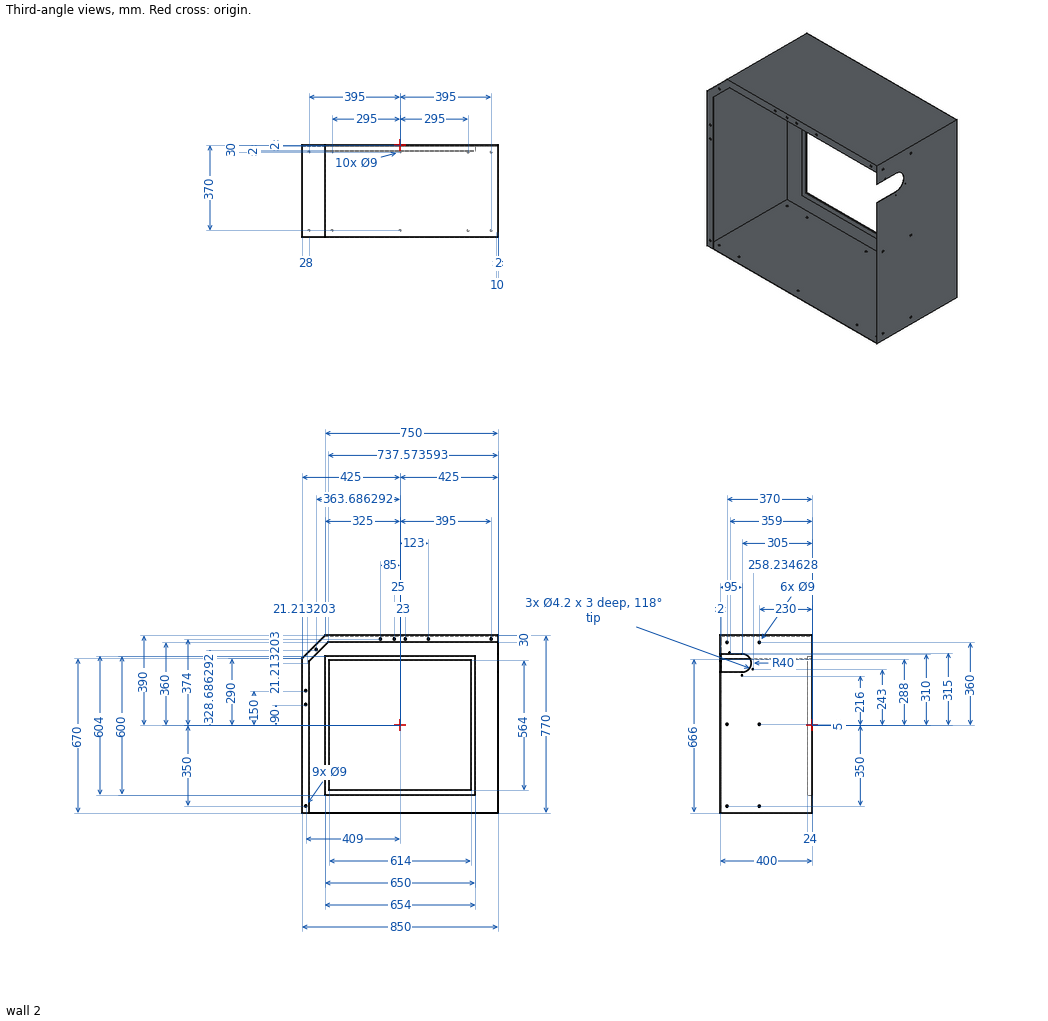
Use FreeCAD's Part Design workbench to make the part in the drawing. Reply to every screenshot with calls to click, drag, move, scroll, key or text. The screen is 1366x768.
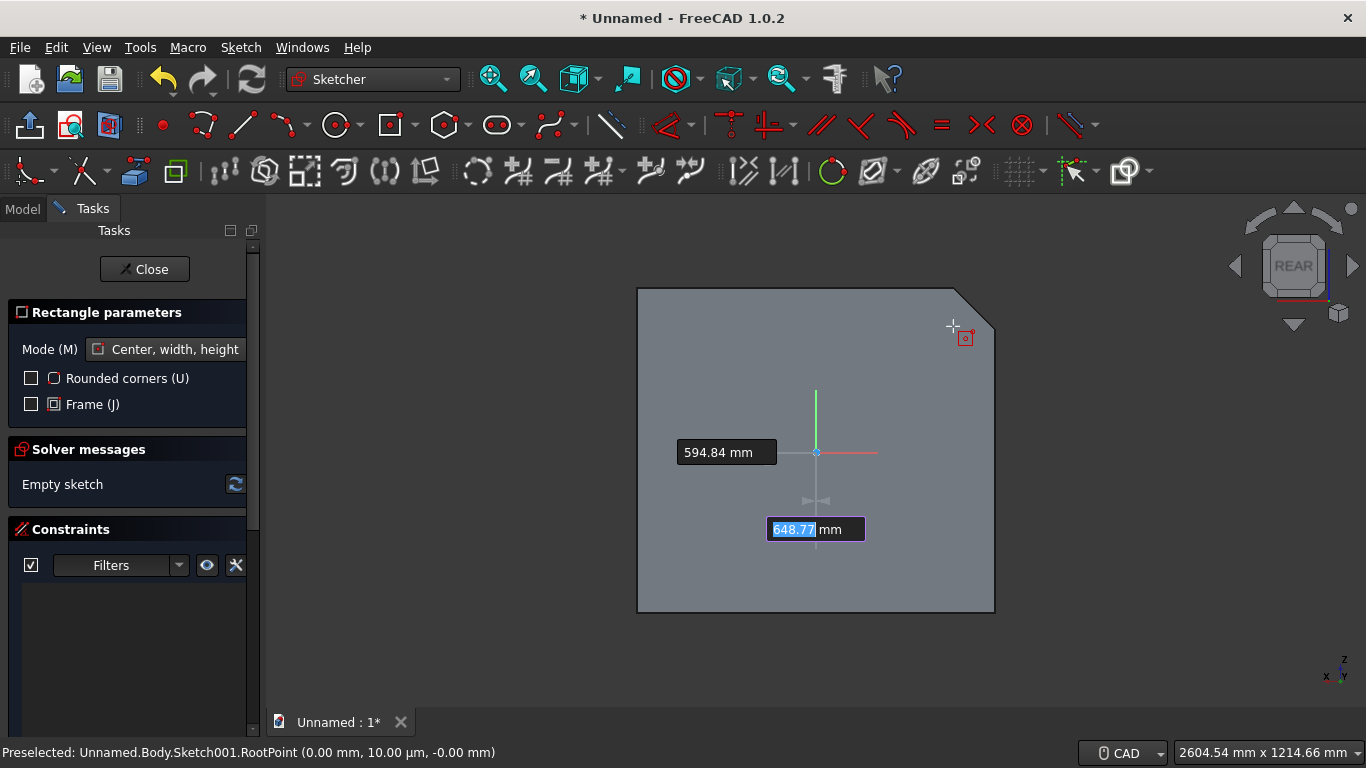
text(650)
key(Tab)
text(600)
key(Return)
key(Escape)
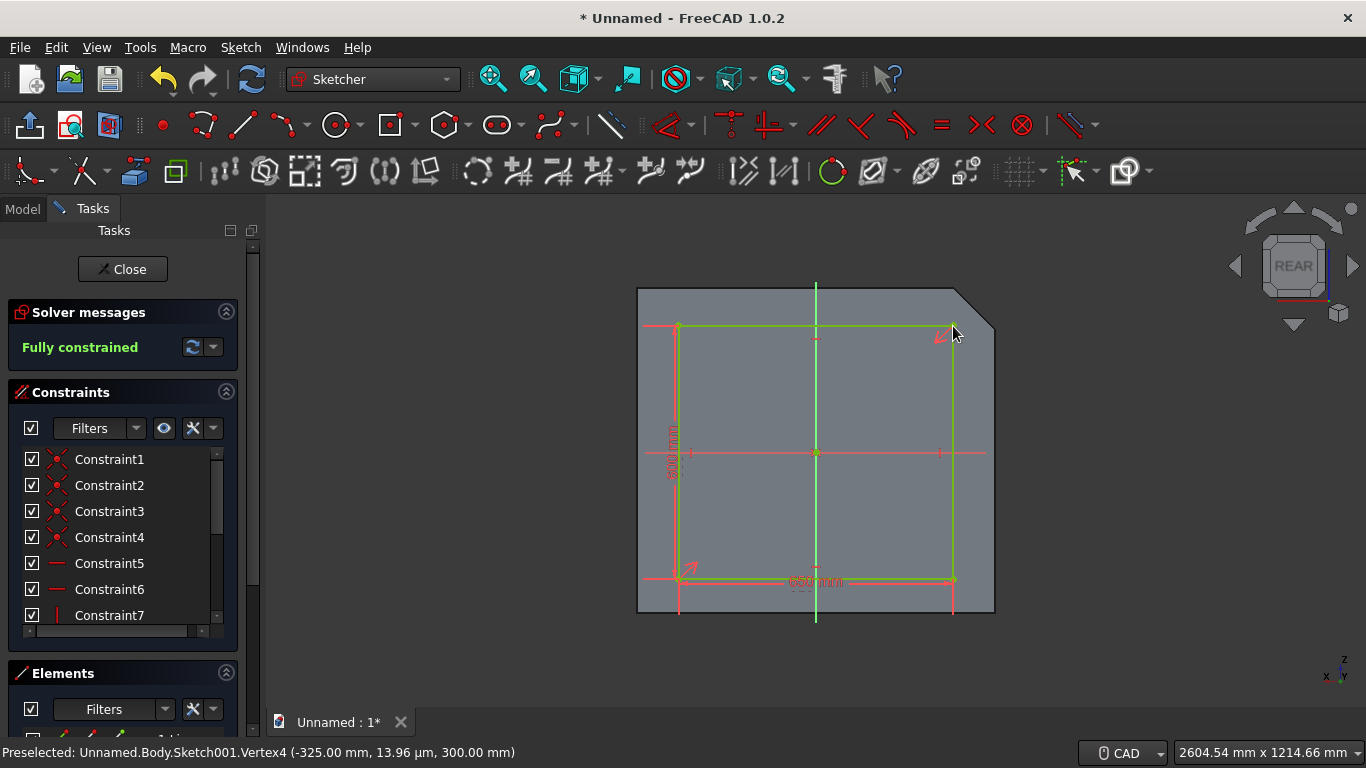
click(123, 269)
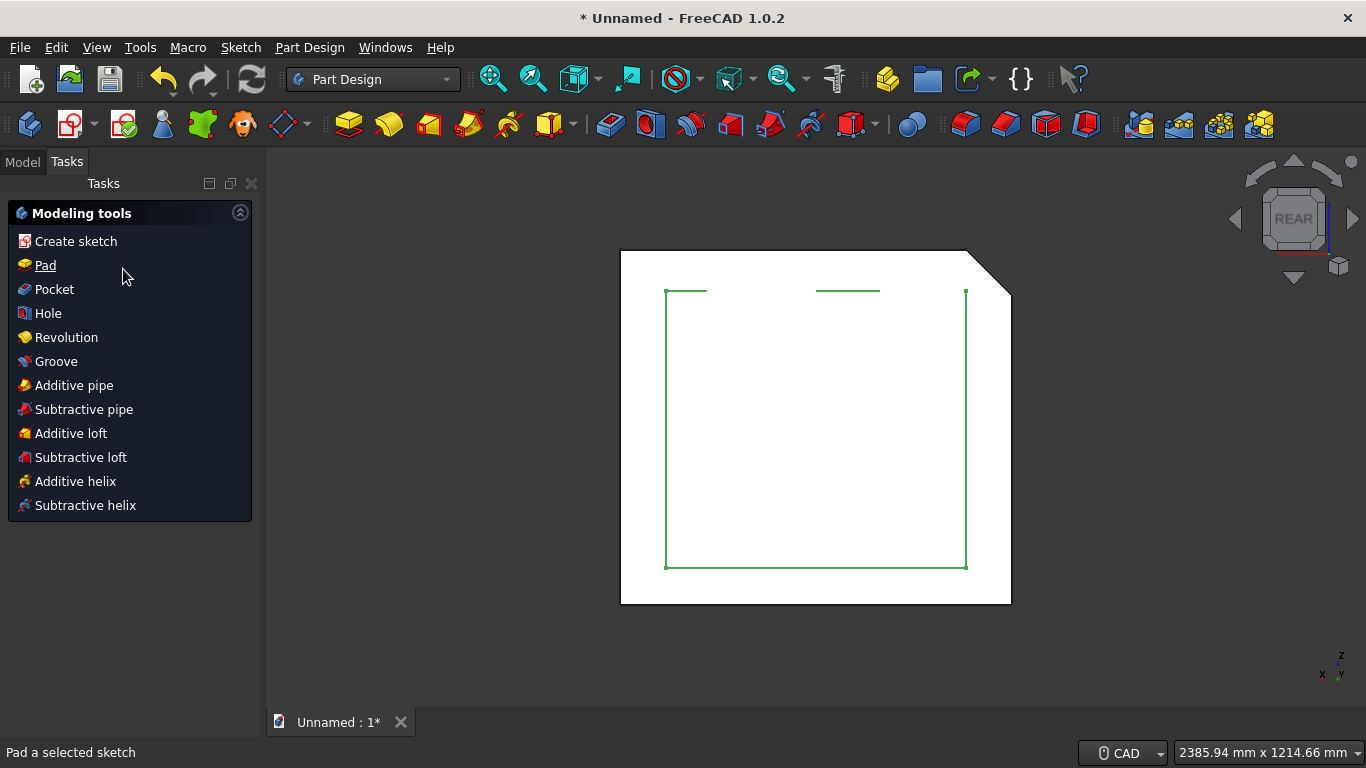
click(612, 124)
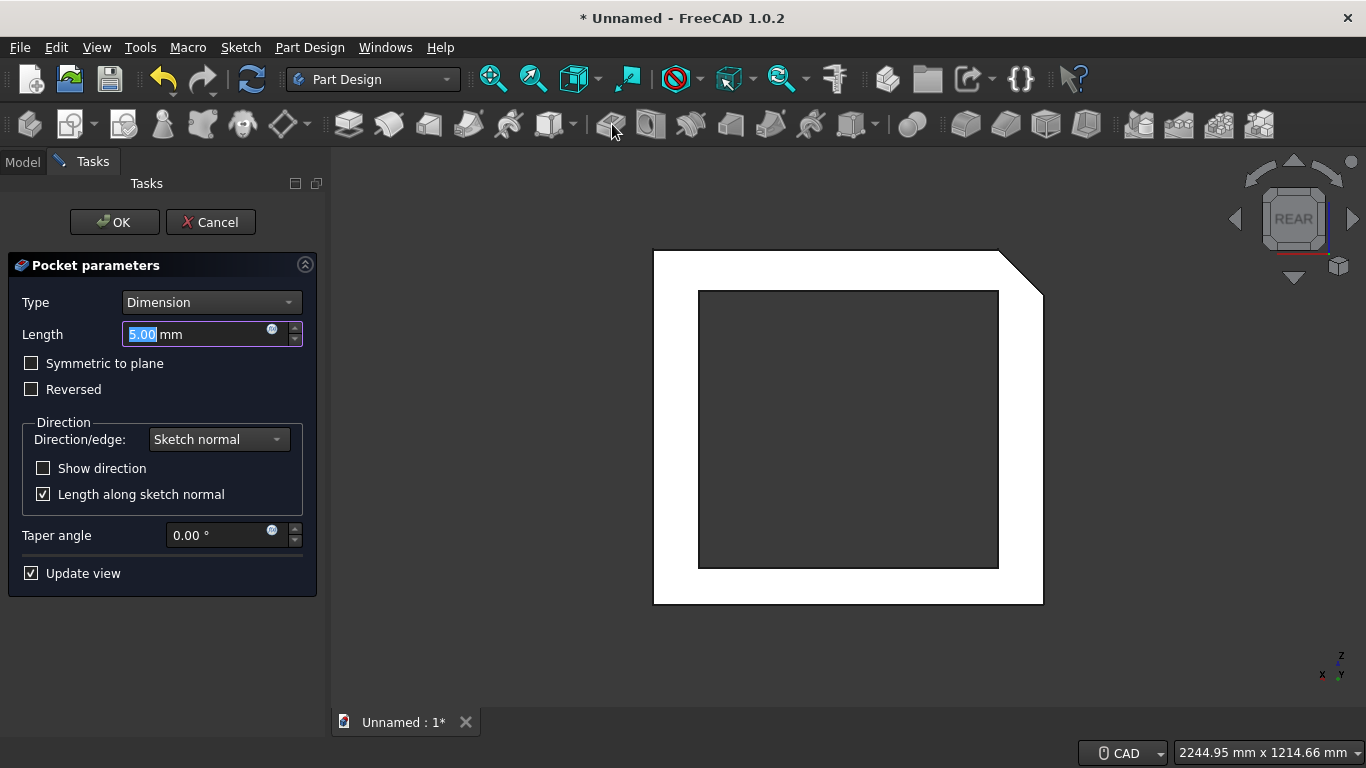
text(2)
key(Tab)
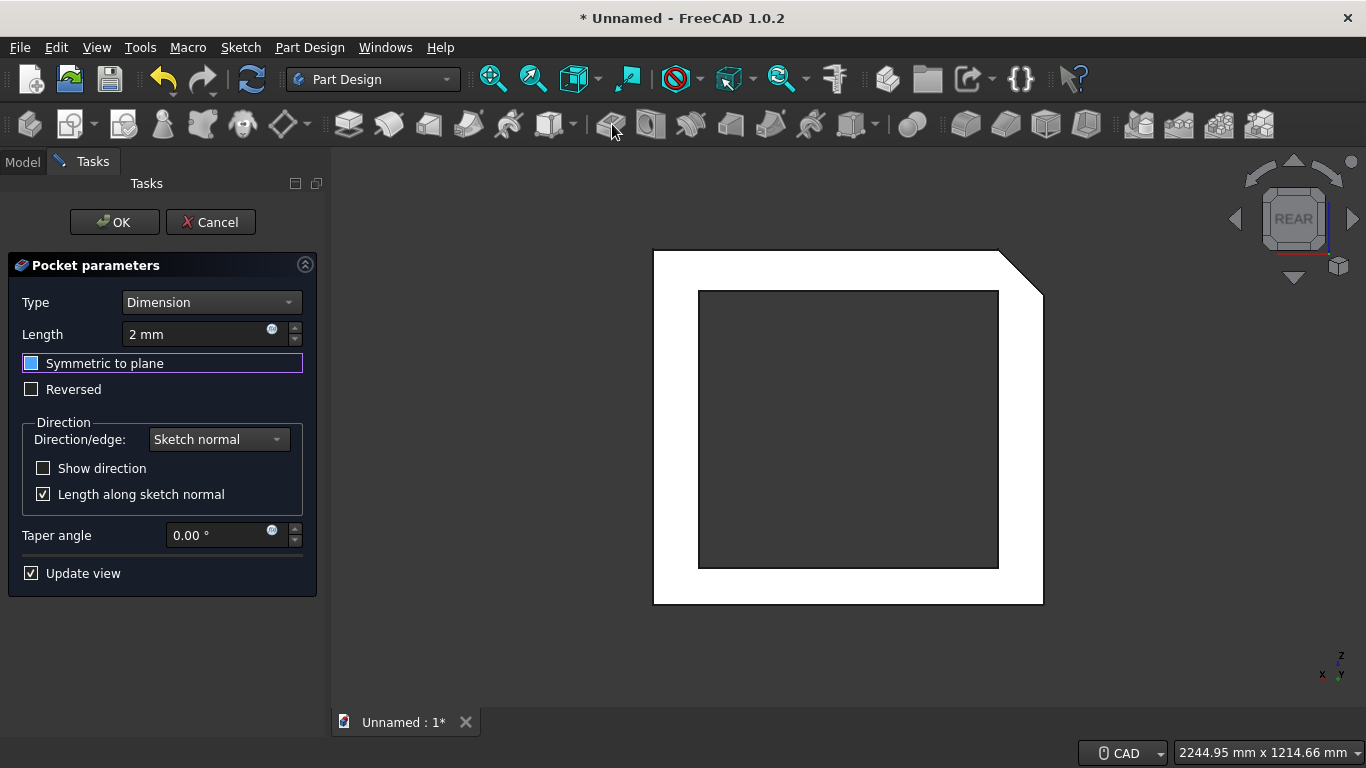
click(115, 222)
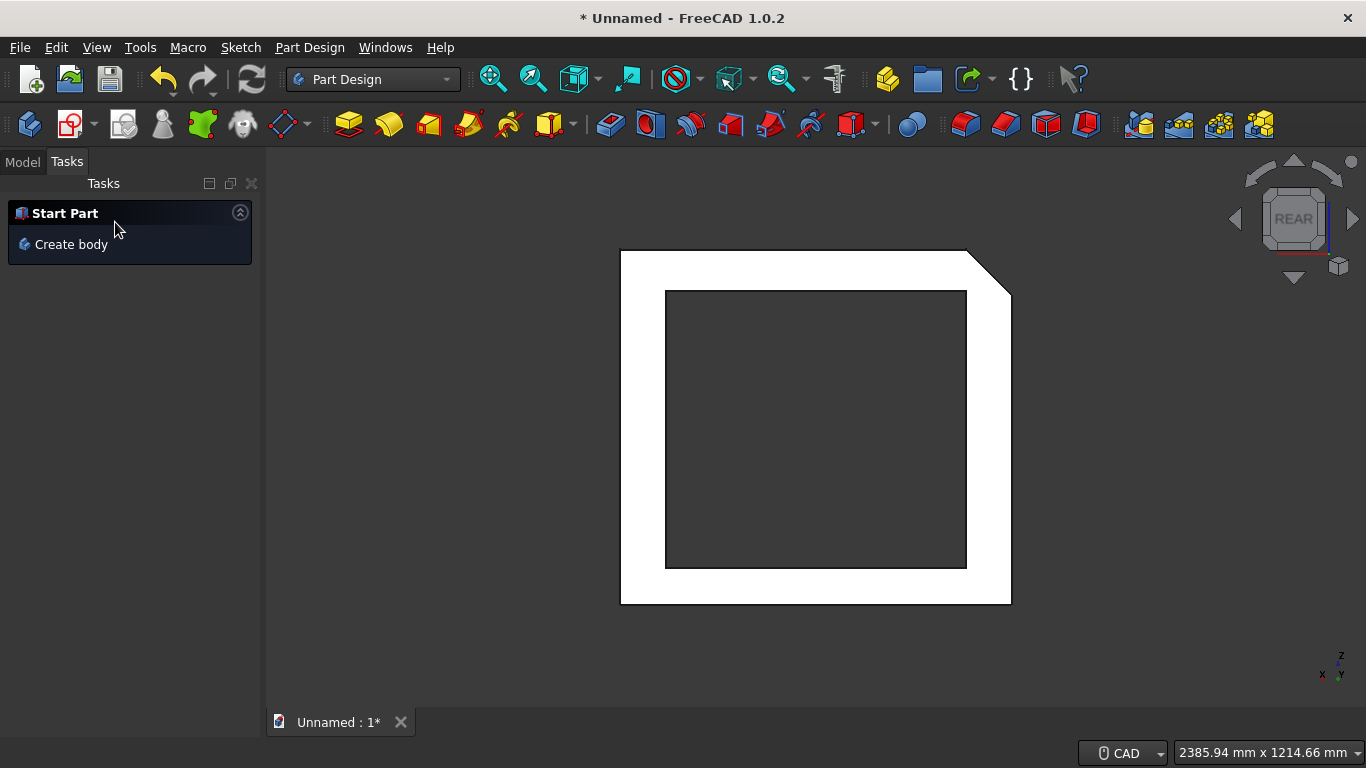
click(648, 274)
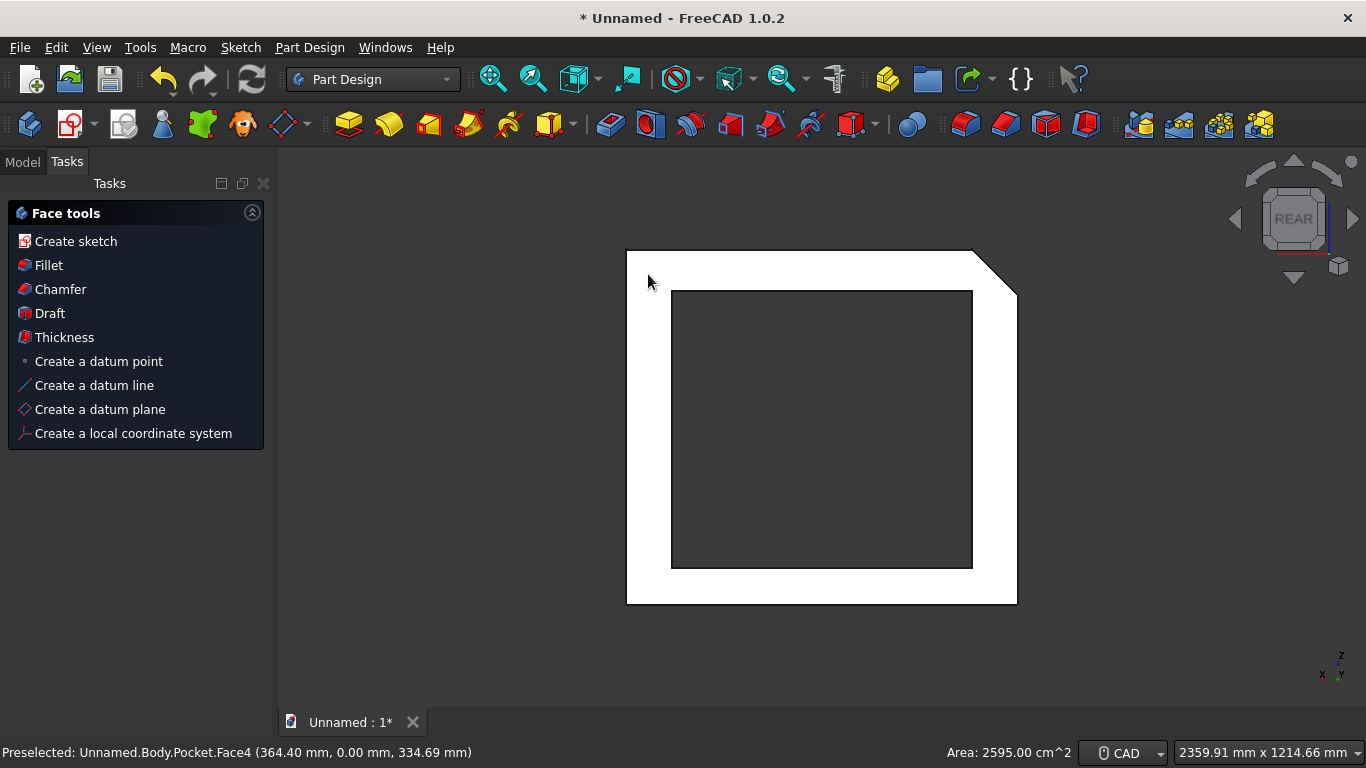
click(70, 124)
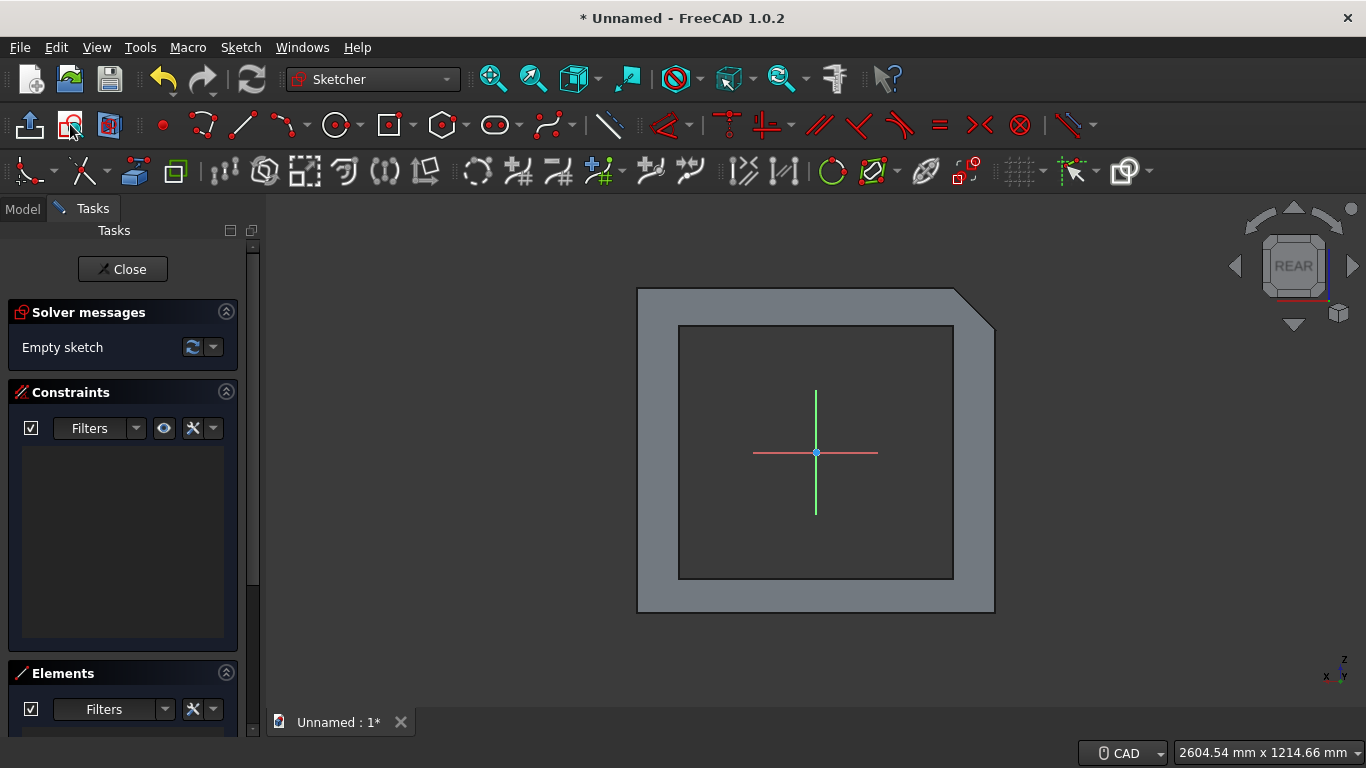
click(390, 126)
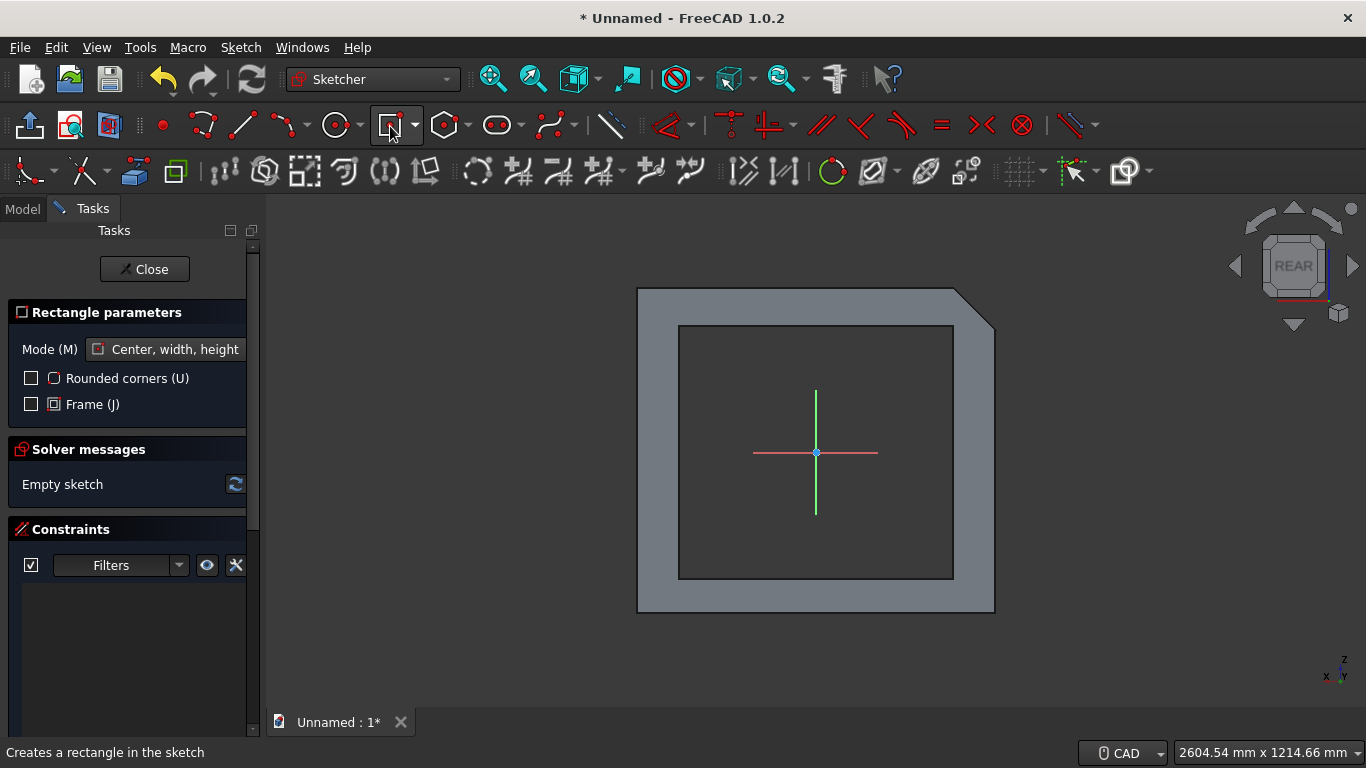
click(816, 453)
move(954, 325)